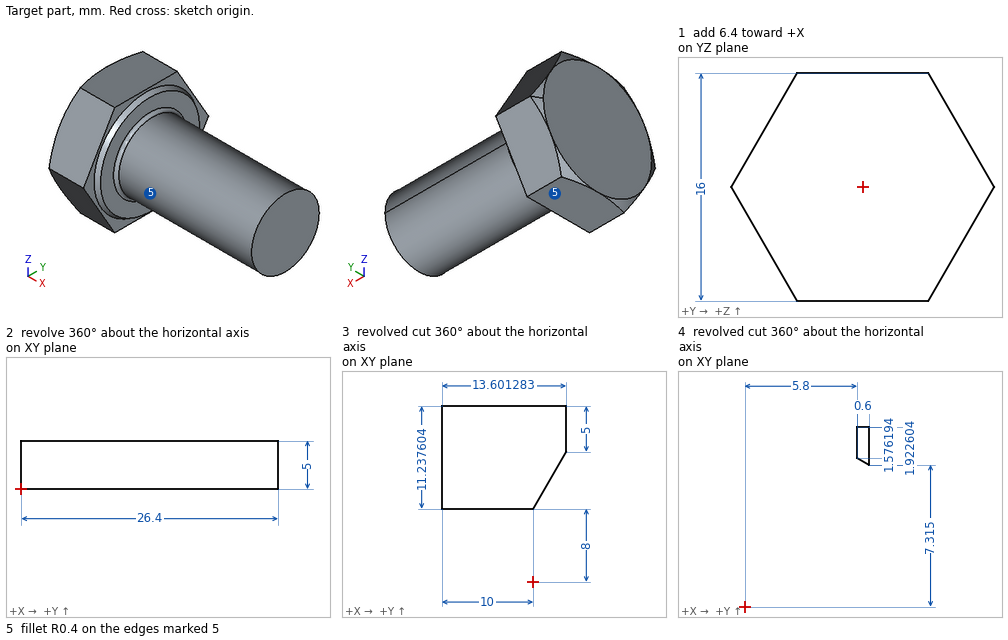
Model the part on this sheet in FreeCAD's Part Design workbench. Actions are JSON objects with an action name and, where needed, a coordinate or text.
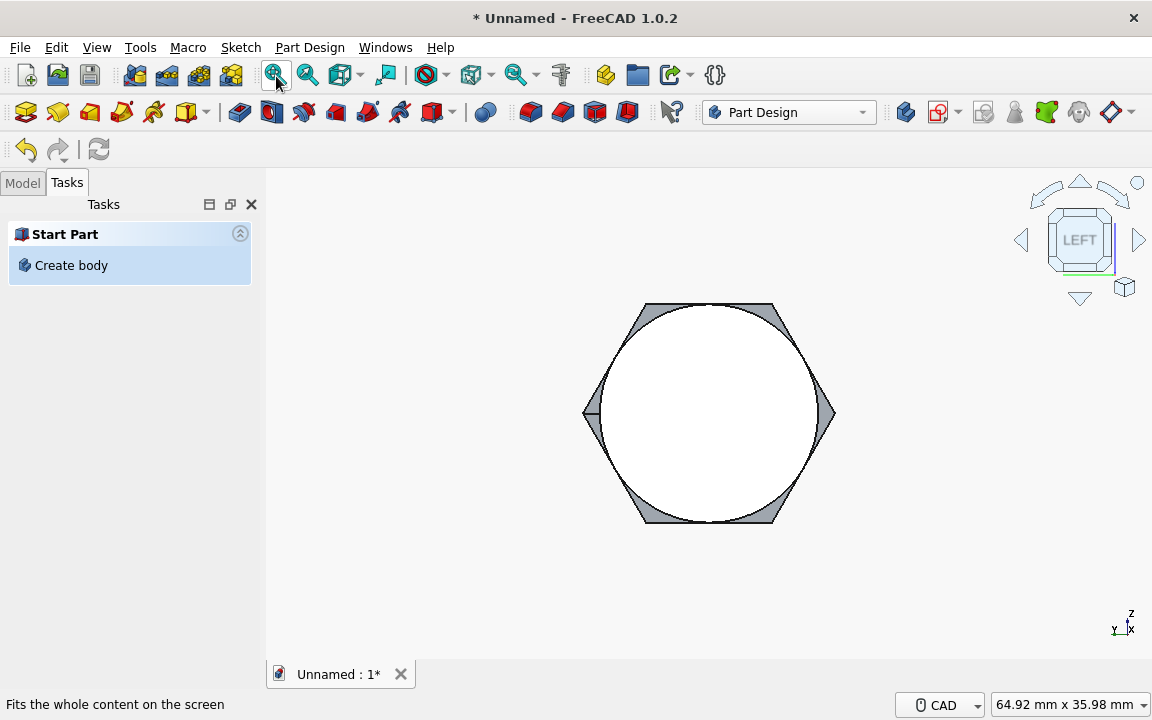
{"action": "key", "text": "v 3"}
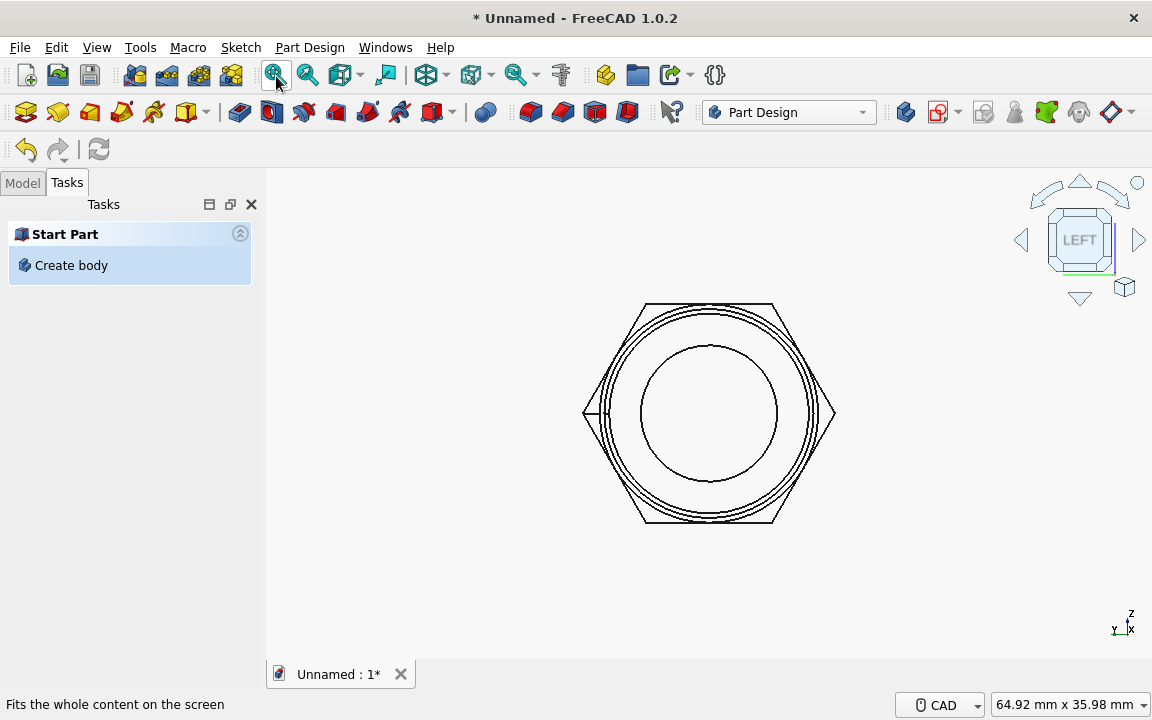
{"action": "key", "text": "0"}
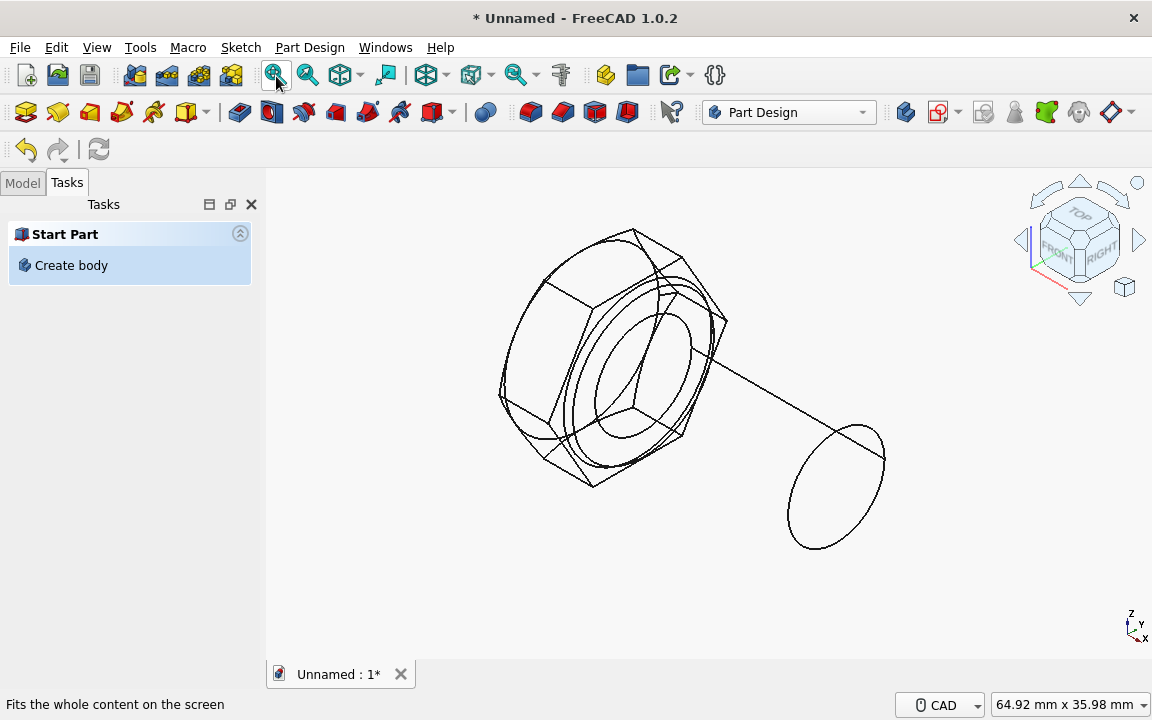
{"action": "left_click", "coordinate": [595, 402]}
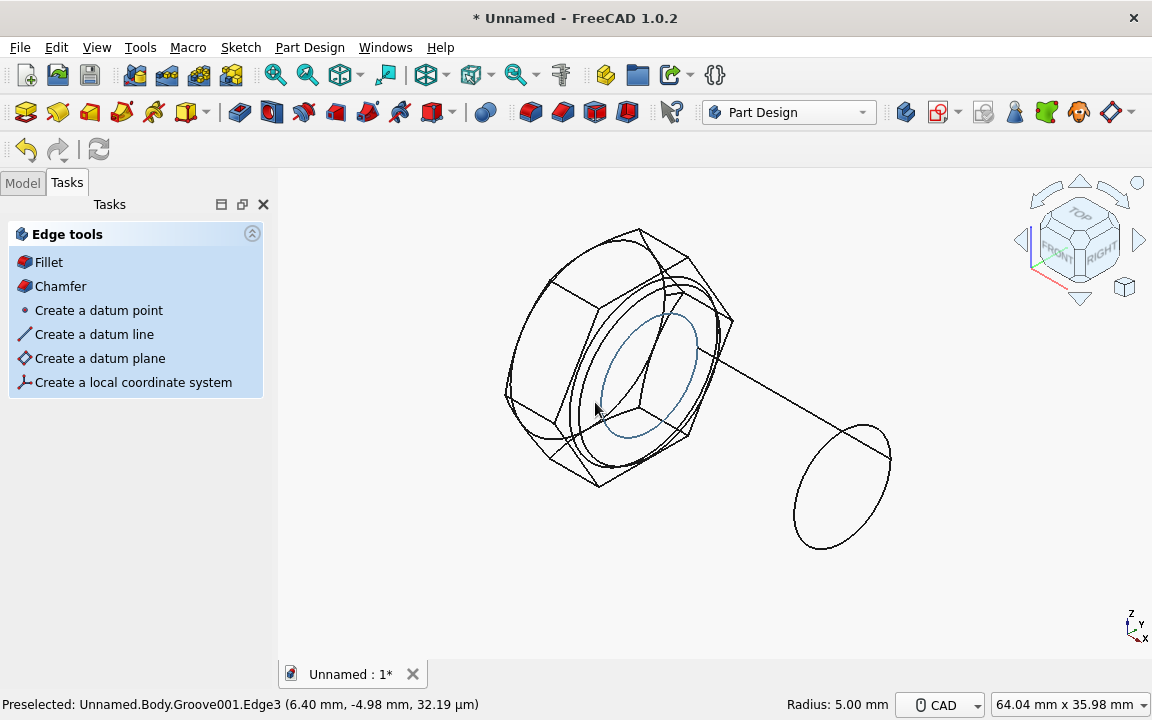
{"action": "key", "text": "v 1"}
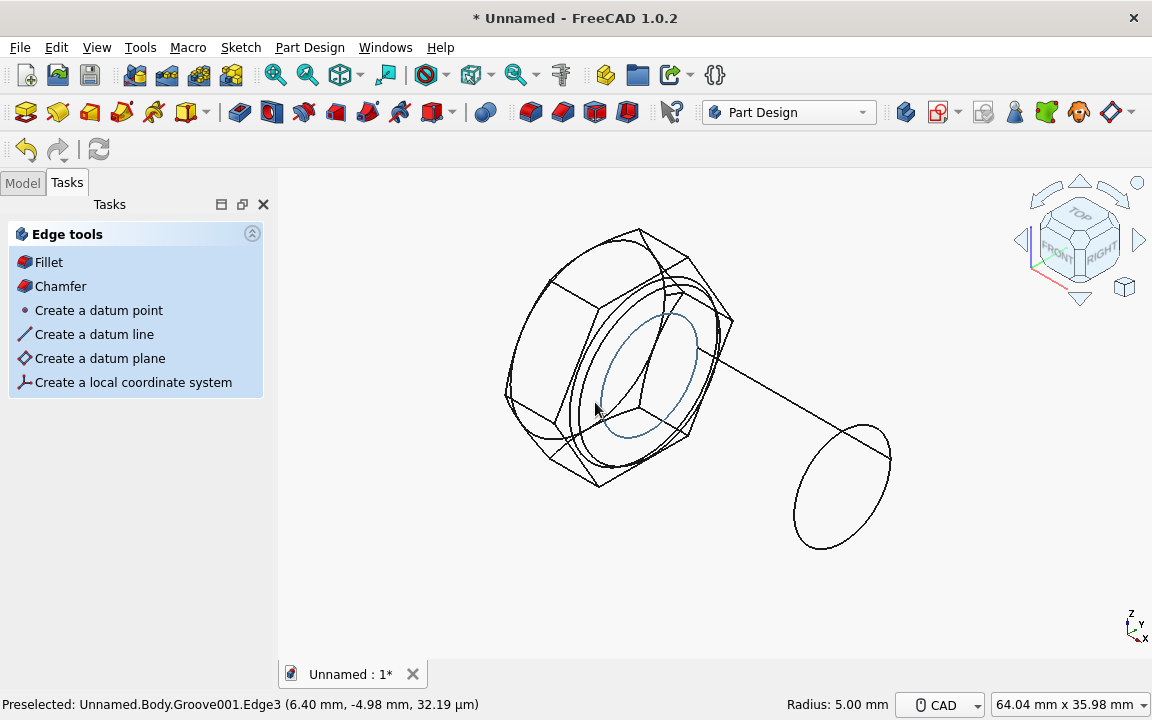
{"action": "left_click", "coordinate": [532, 112]}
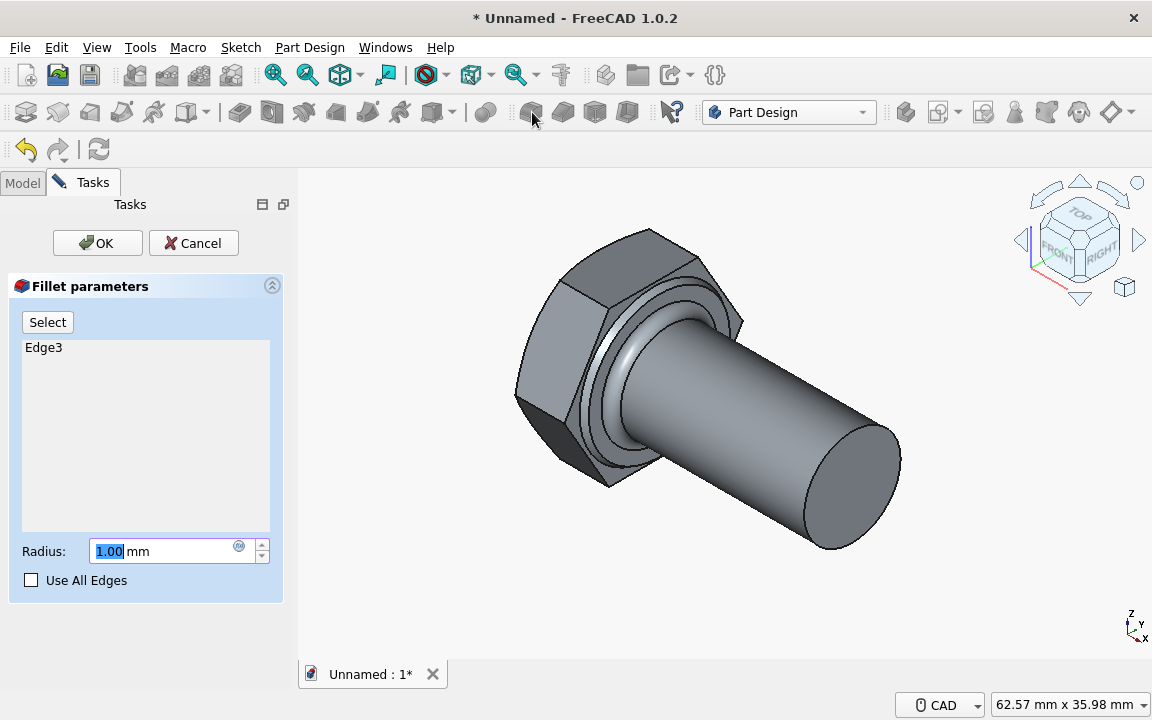
{"action": "type", "text": "0.4"}
{"action": "key", "text": "Tab"}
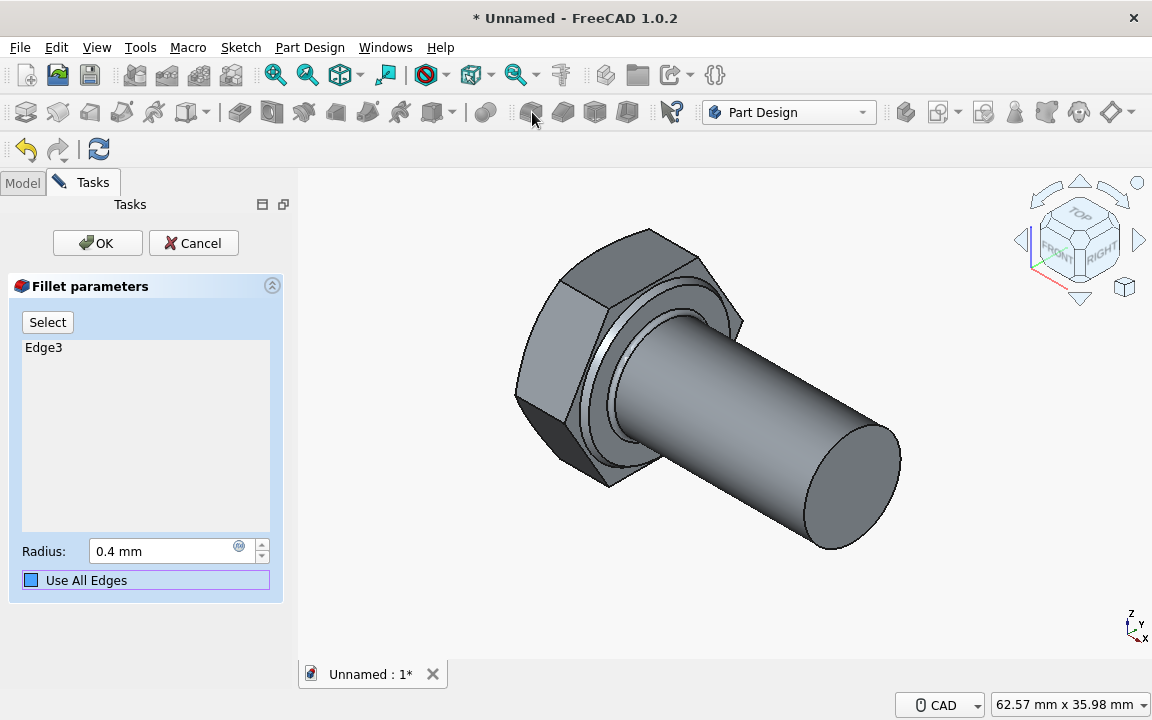
{"action": "left_click", "coordinate": [98, 243]}